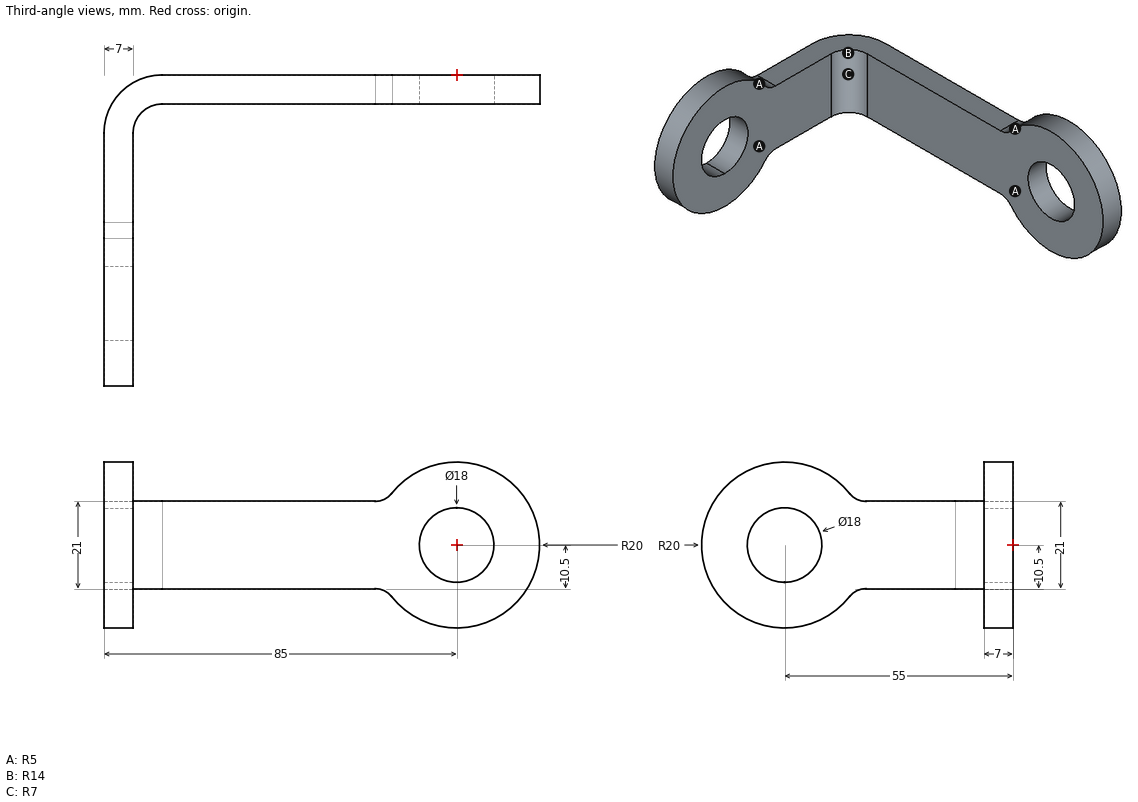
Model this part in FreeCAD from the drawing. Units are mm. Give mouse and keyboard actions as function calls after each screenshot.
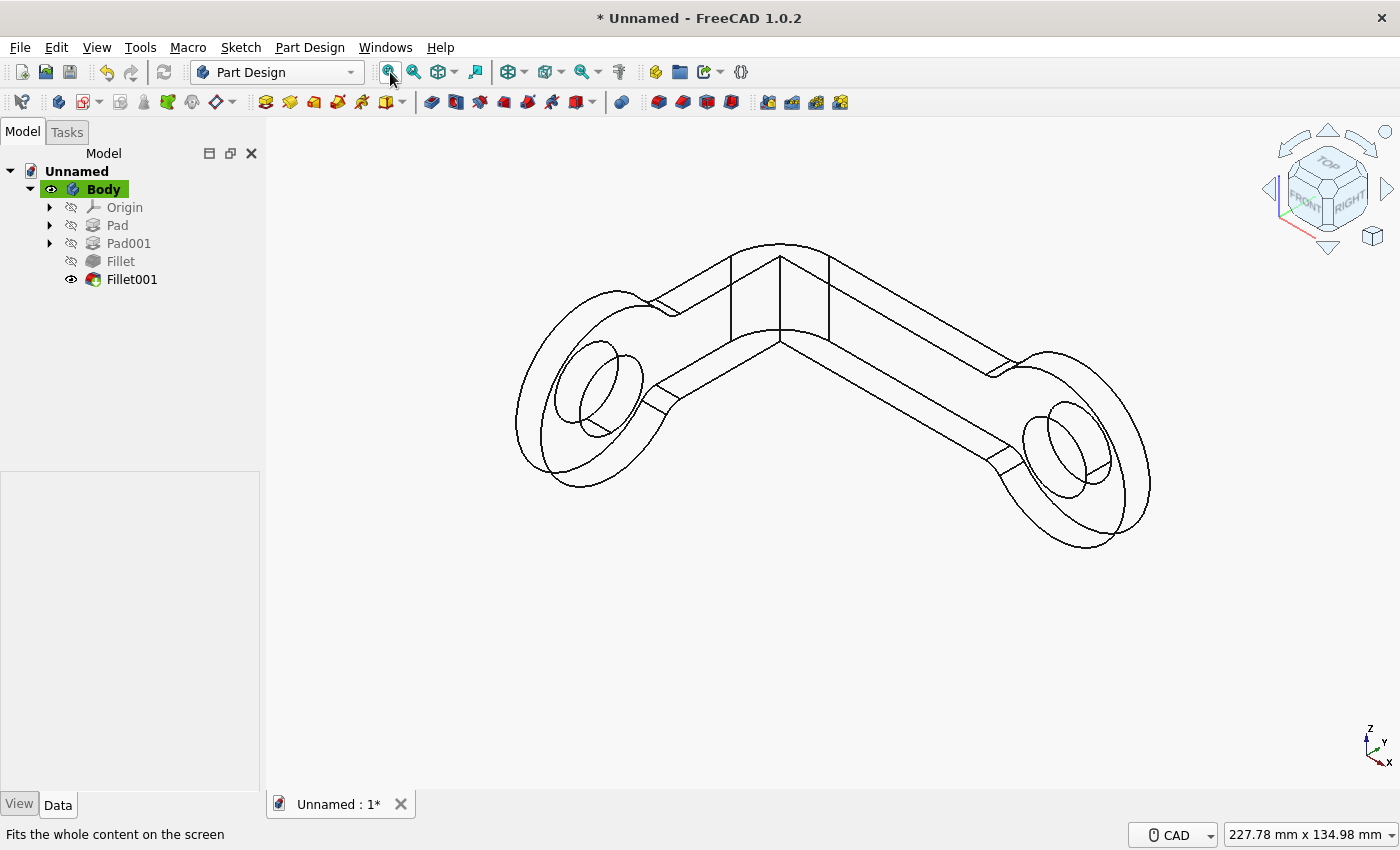
click(780, 298)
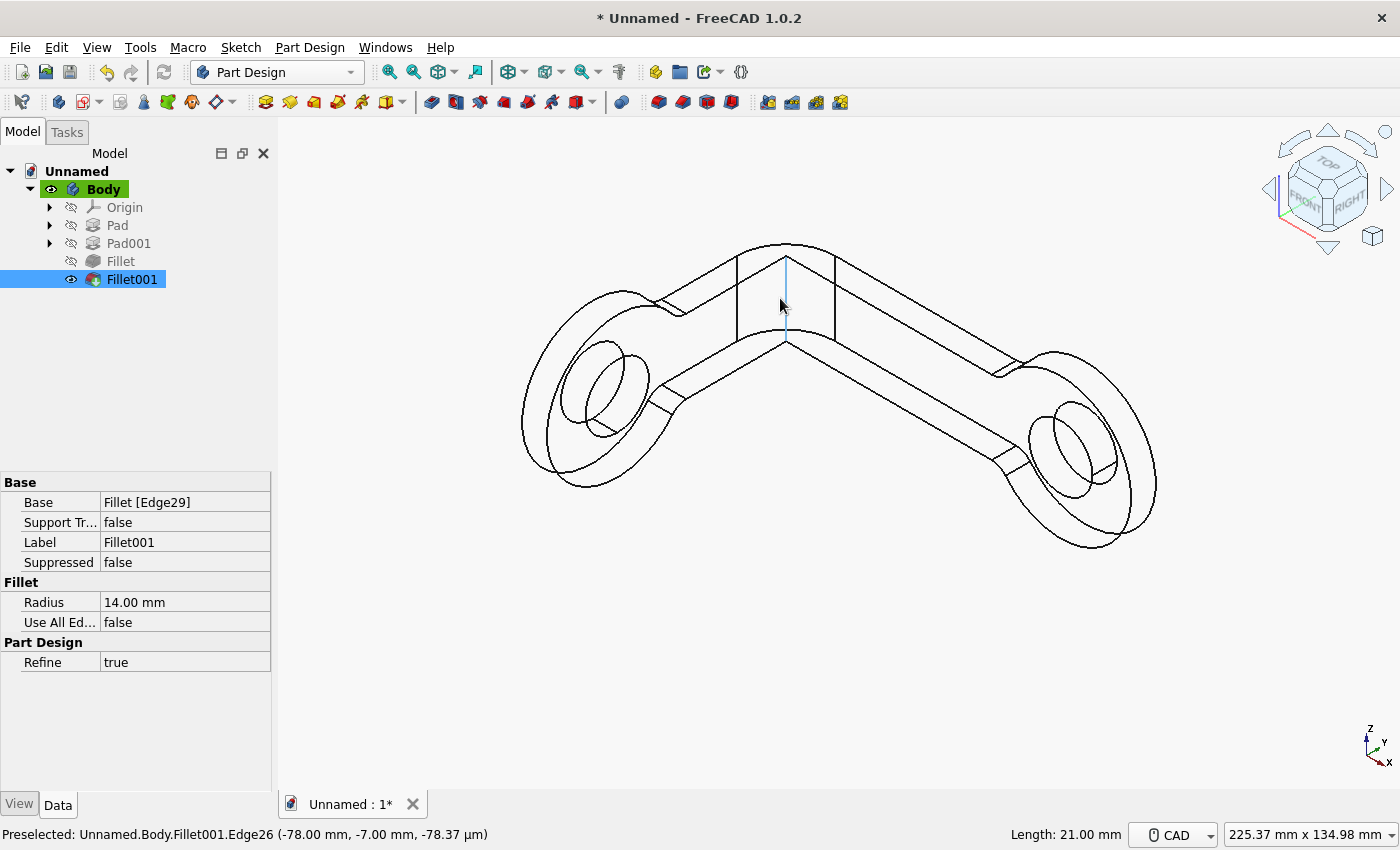
key(v)
key(1)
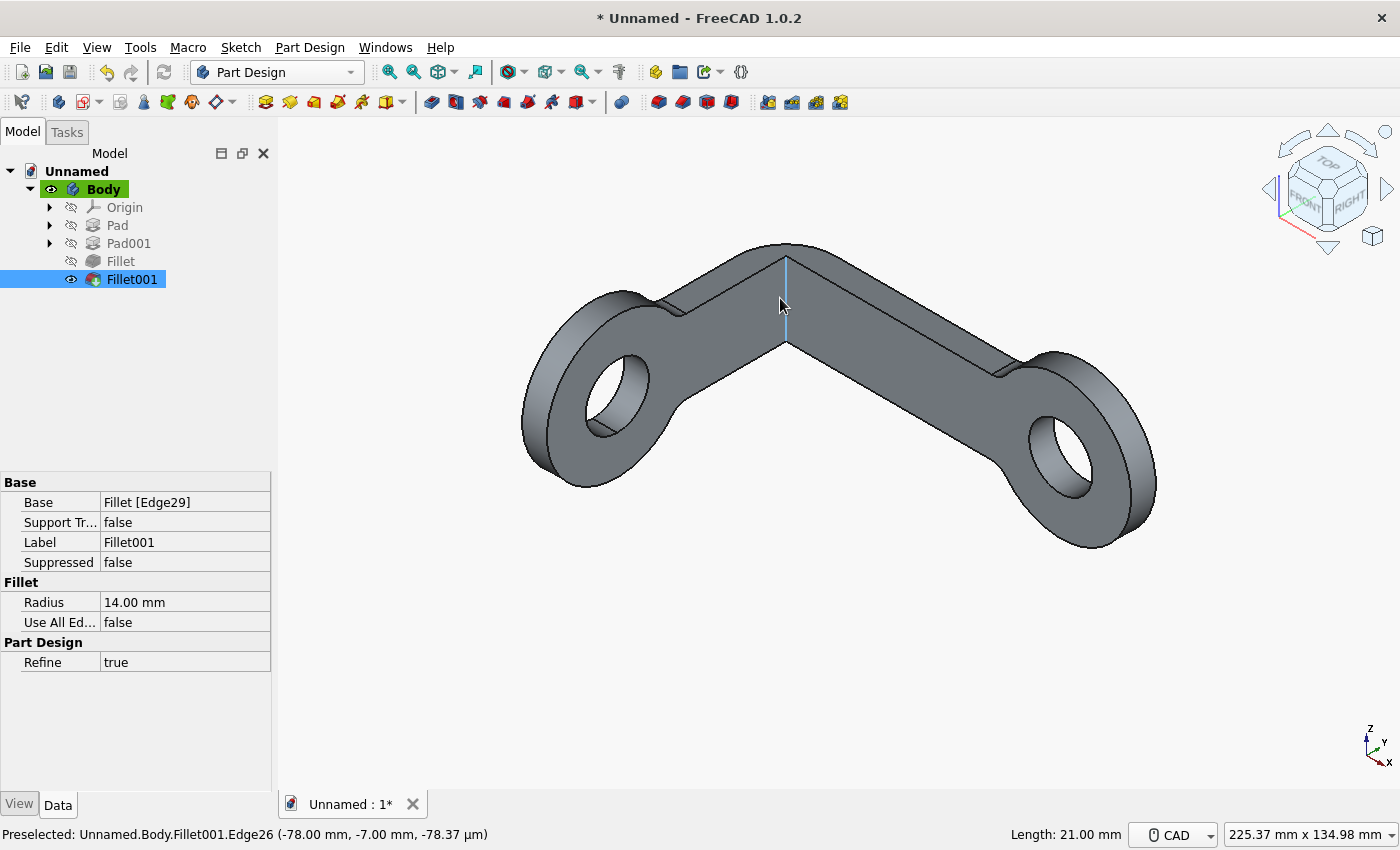
click(660, 102)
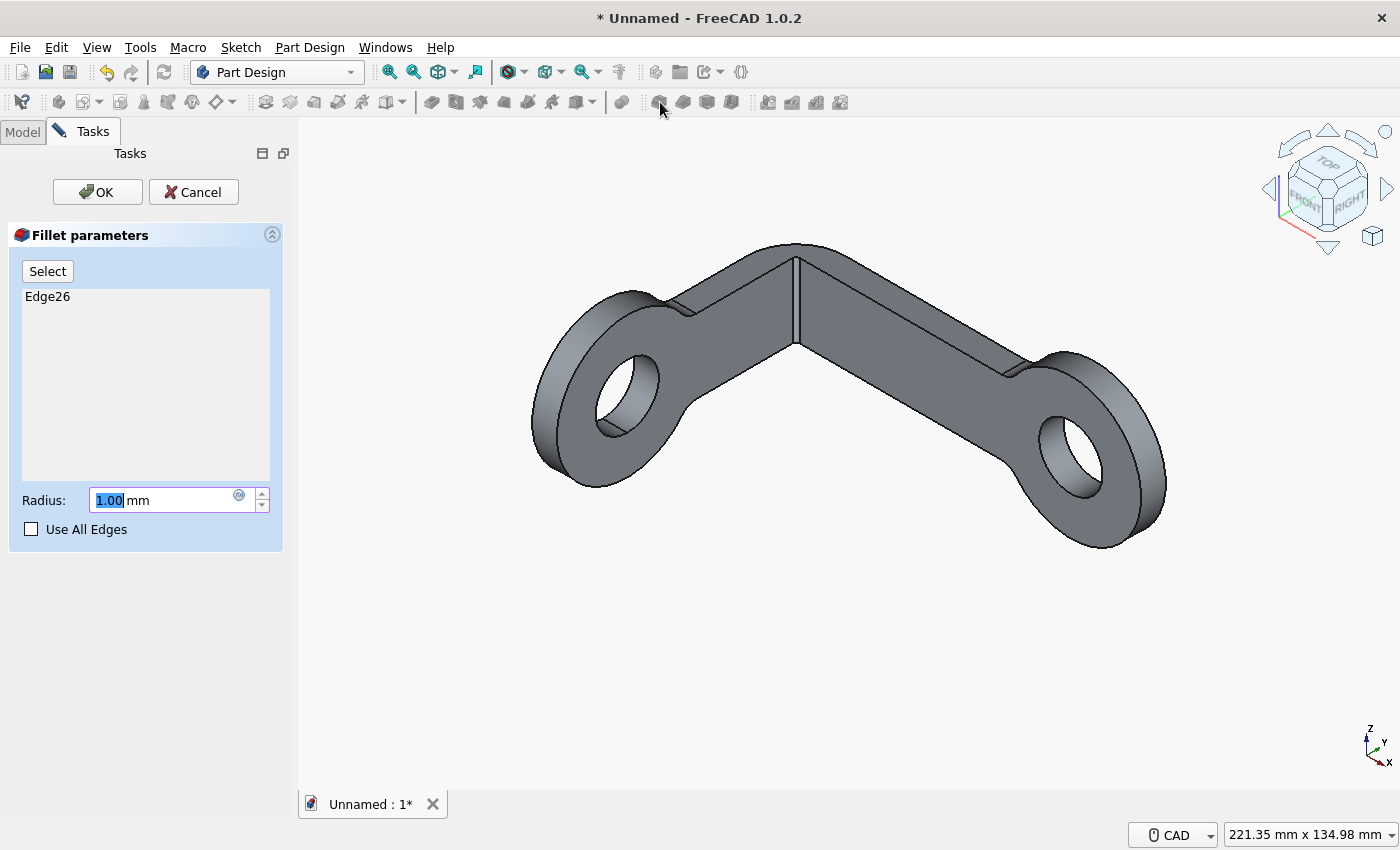
text(7)
key(Tab)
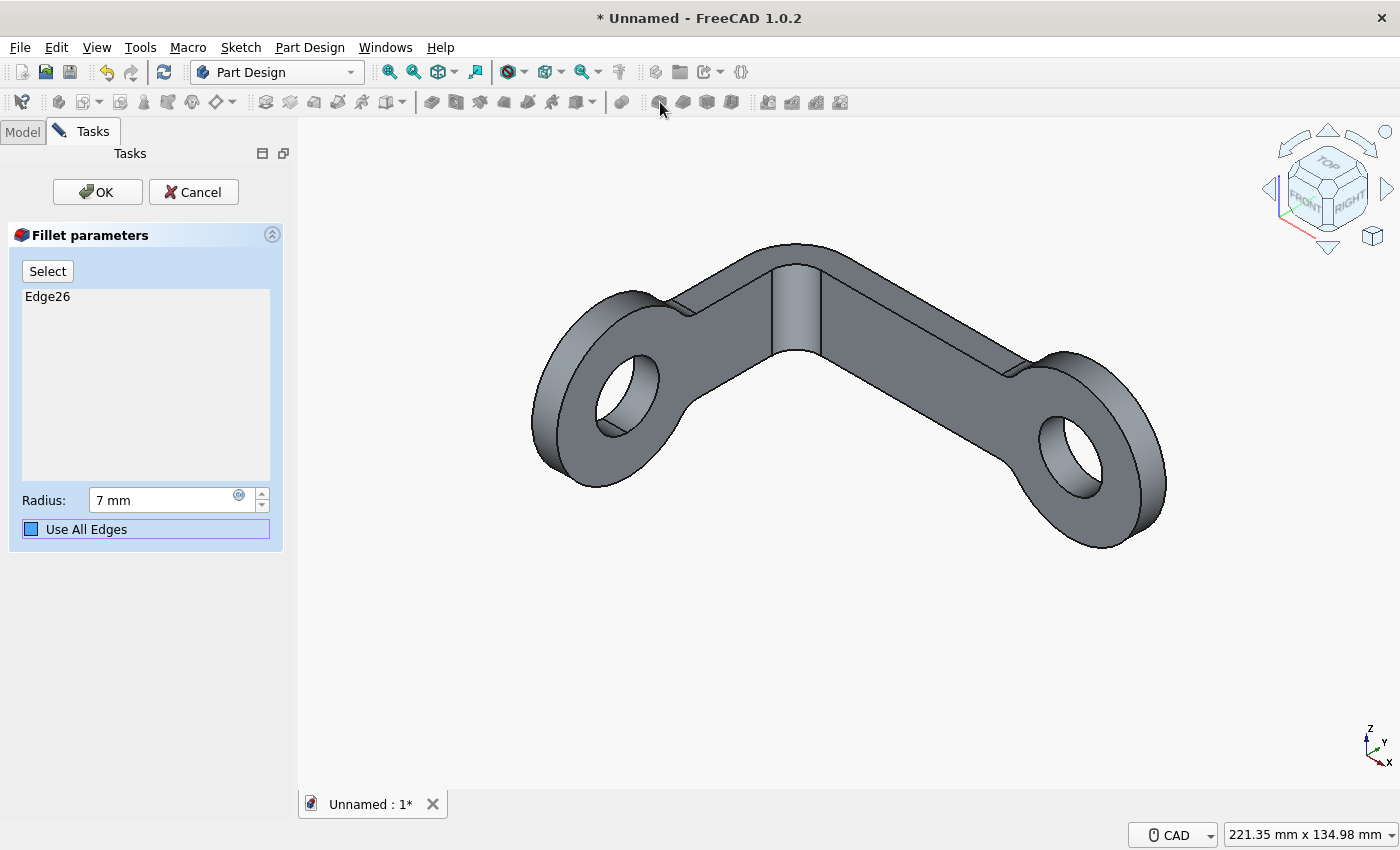
click(98, 192)